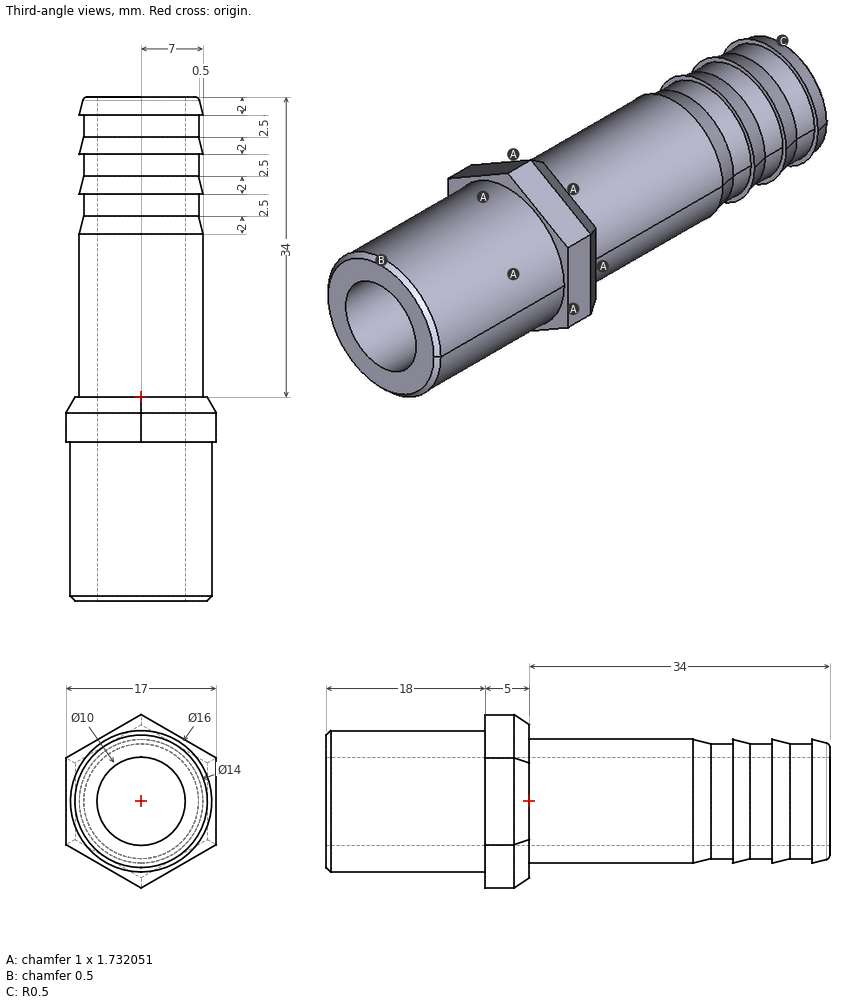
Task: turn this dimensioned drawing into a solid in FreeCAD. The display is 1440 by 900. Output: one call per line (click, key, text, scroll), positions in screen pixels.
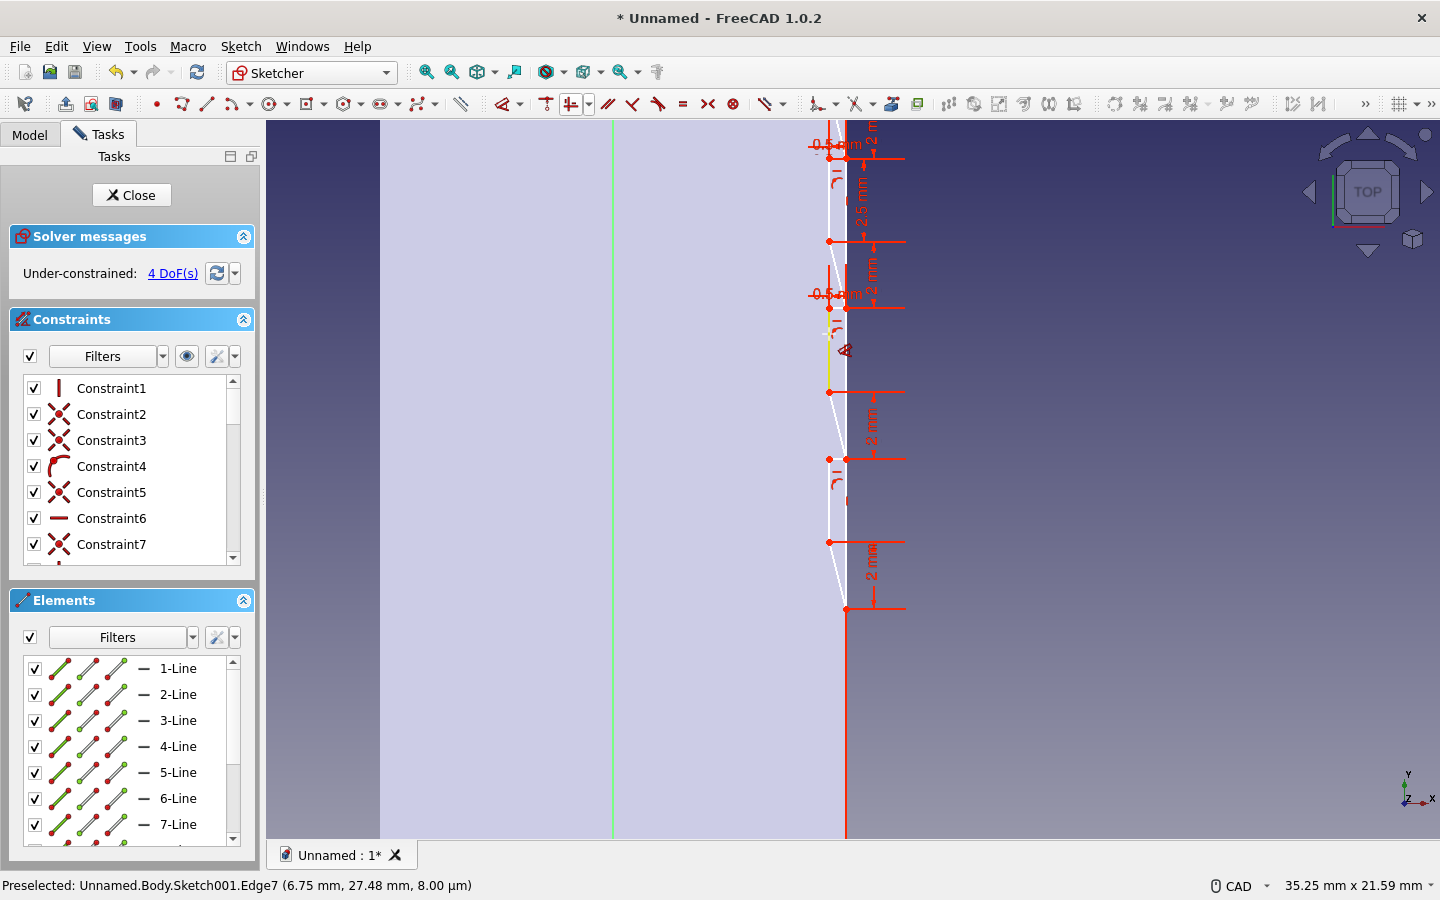
click(829, 334)
click(863, 350)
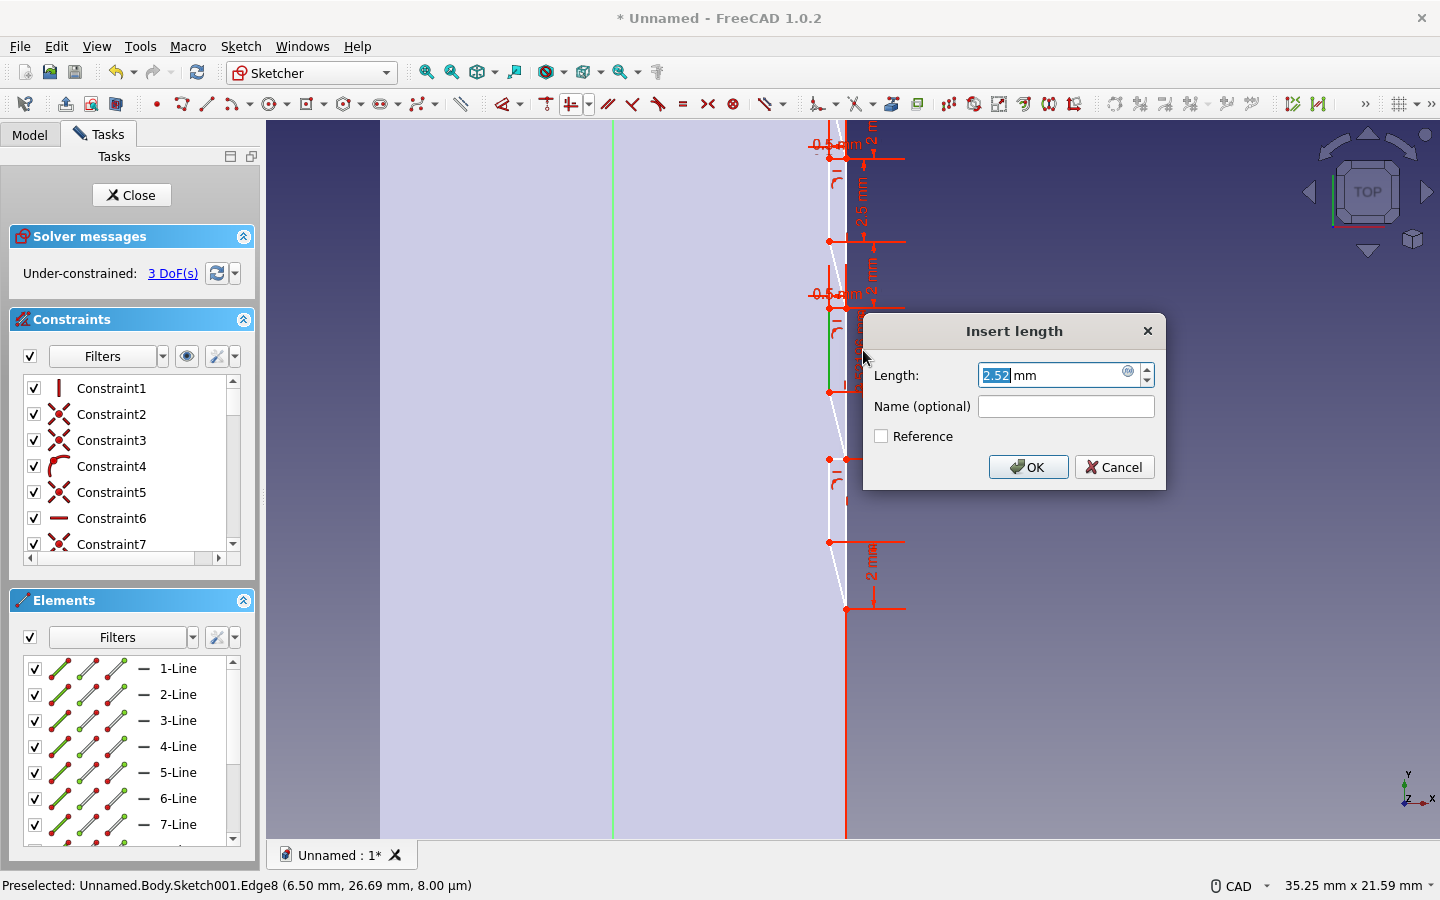
text(2.5)
key(Return)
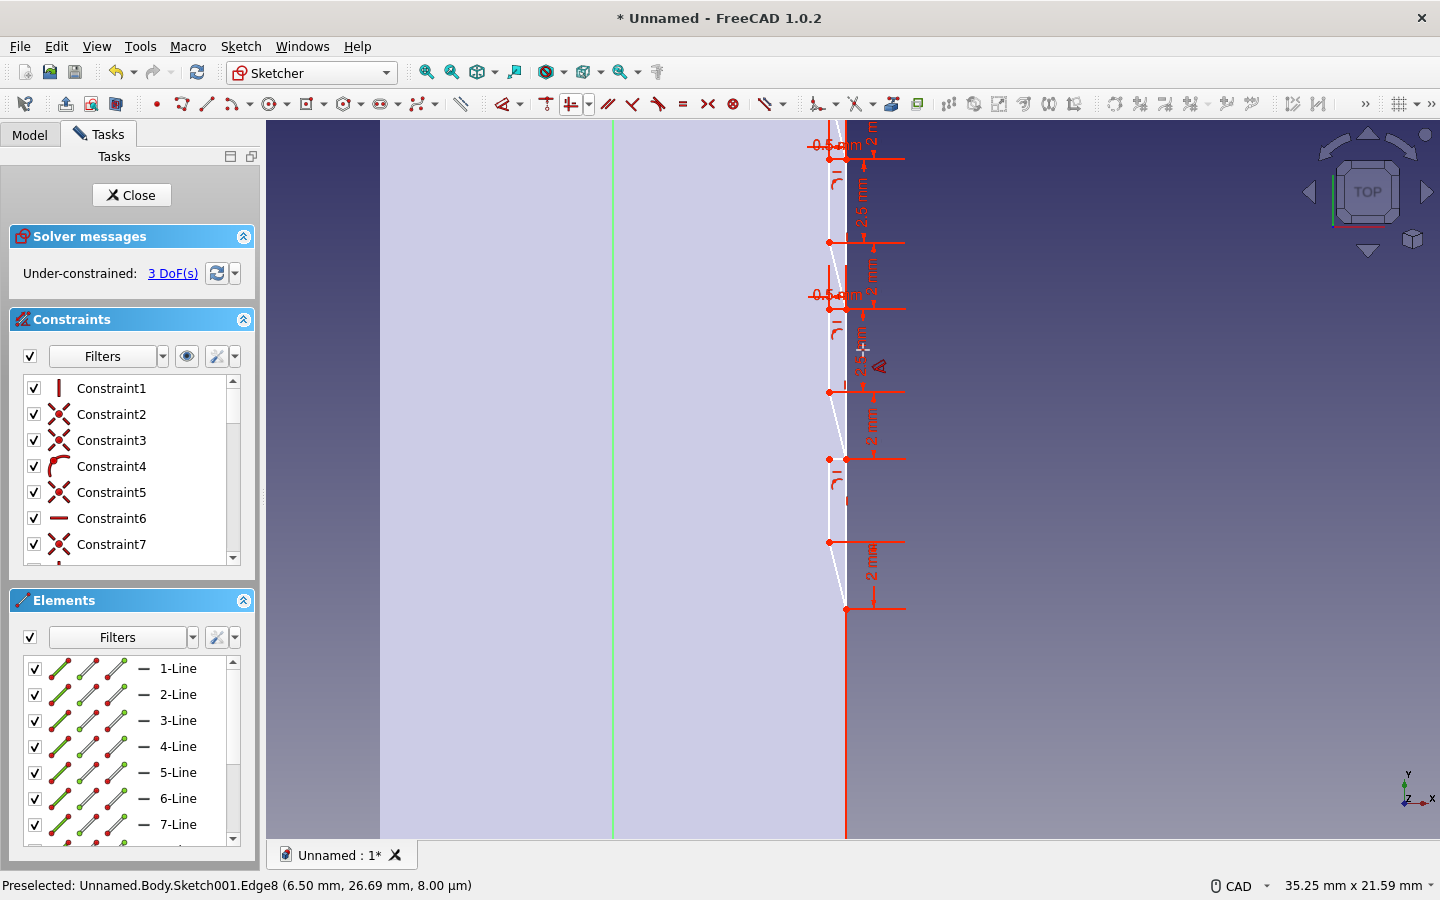
scroll(838, 459, up, 5)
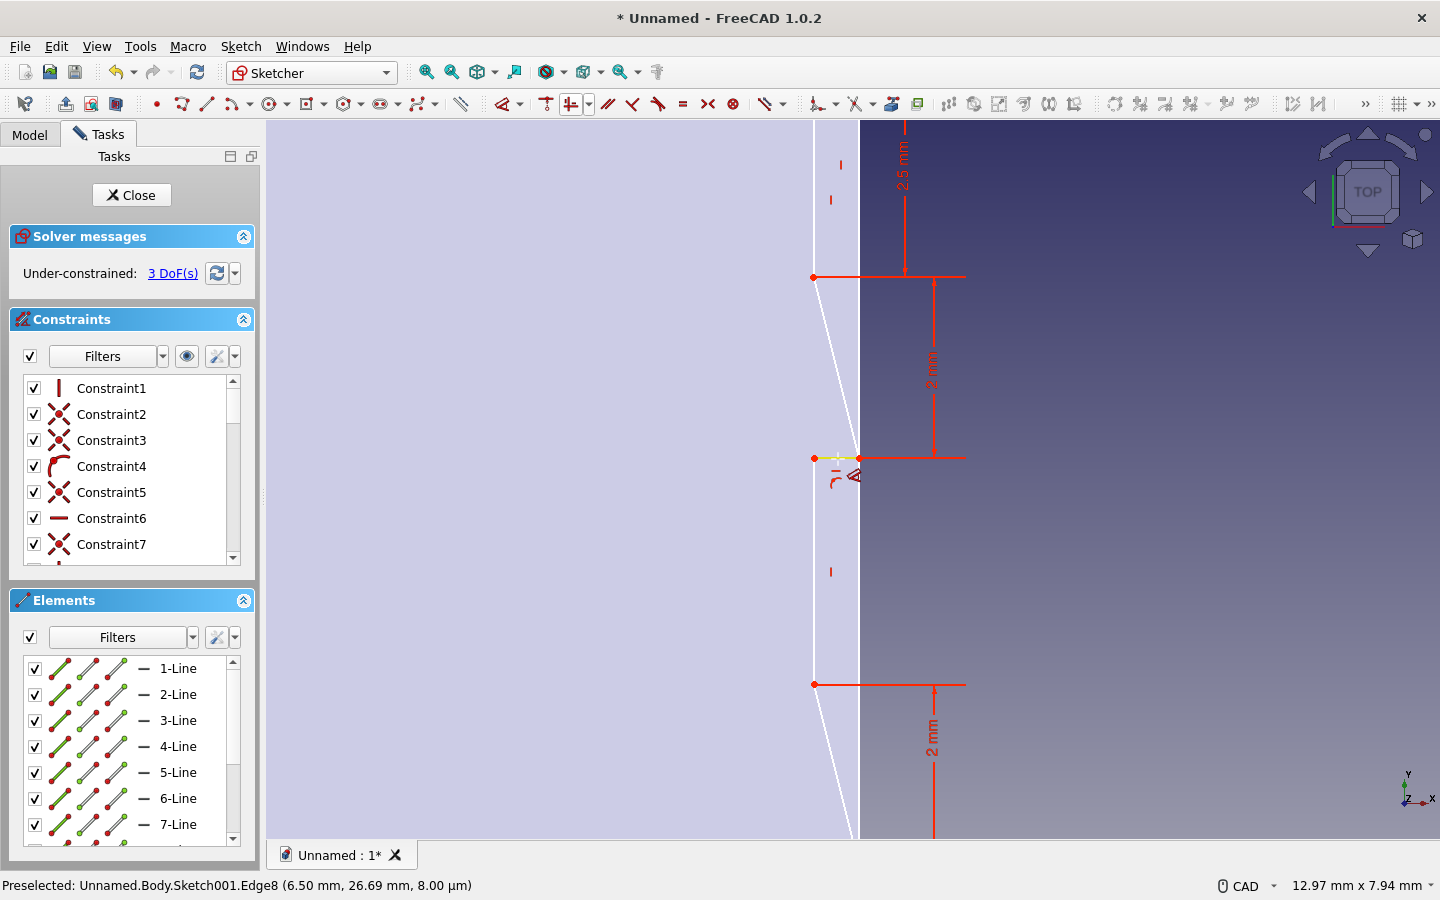
click(837, 458)
click(837, 424)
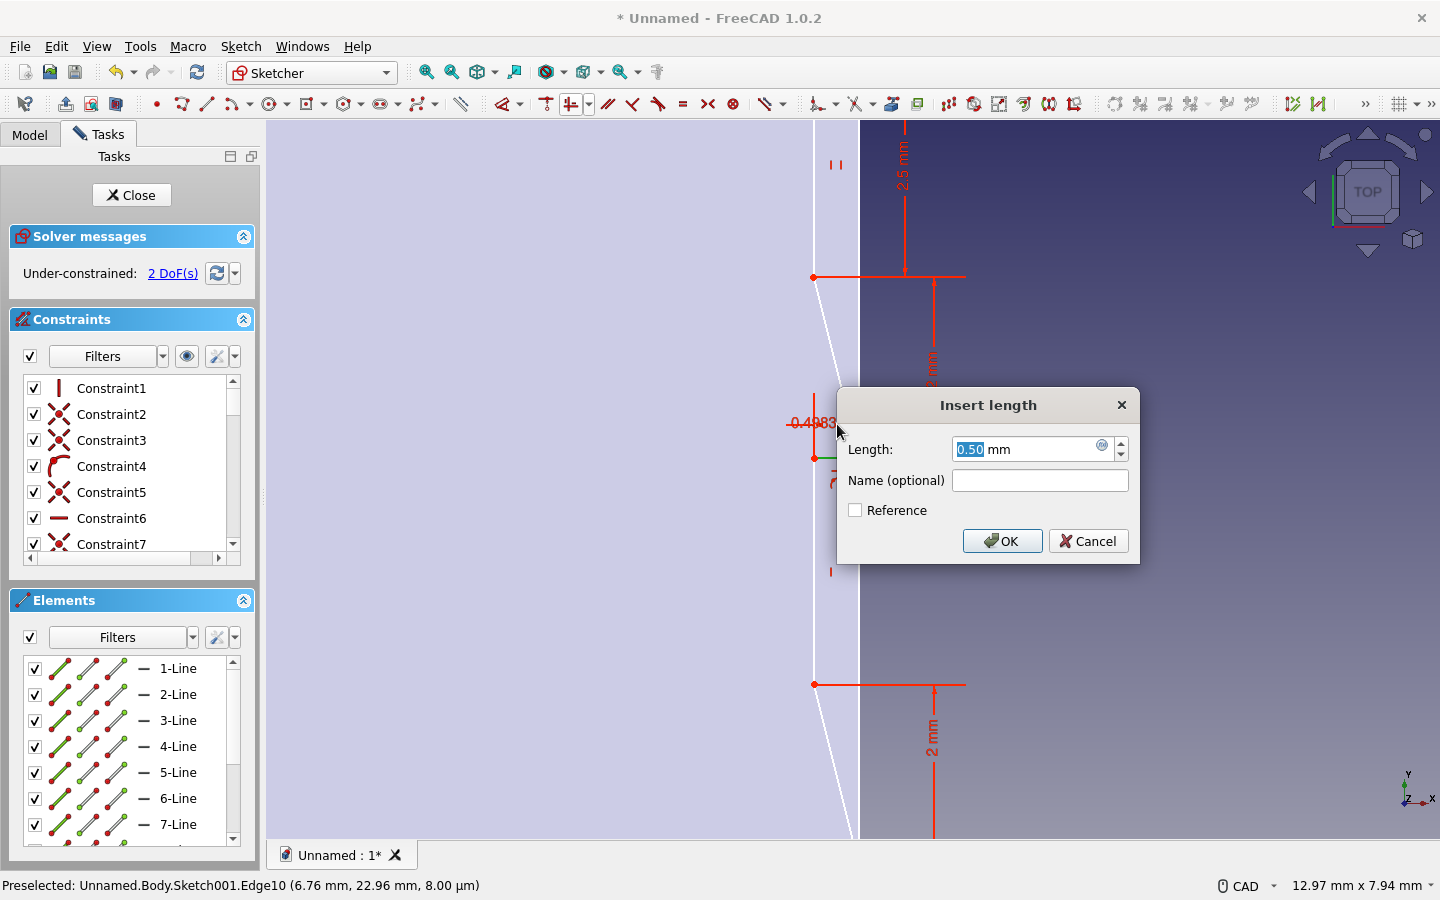
text(0.5)
key(Return)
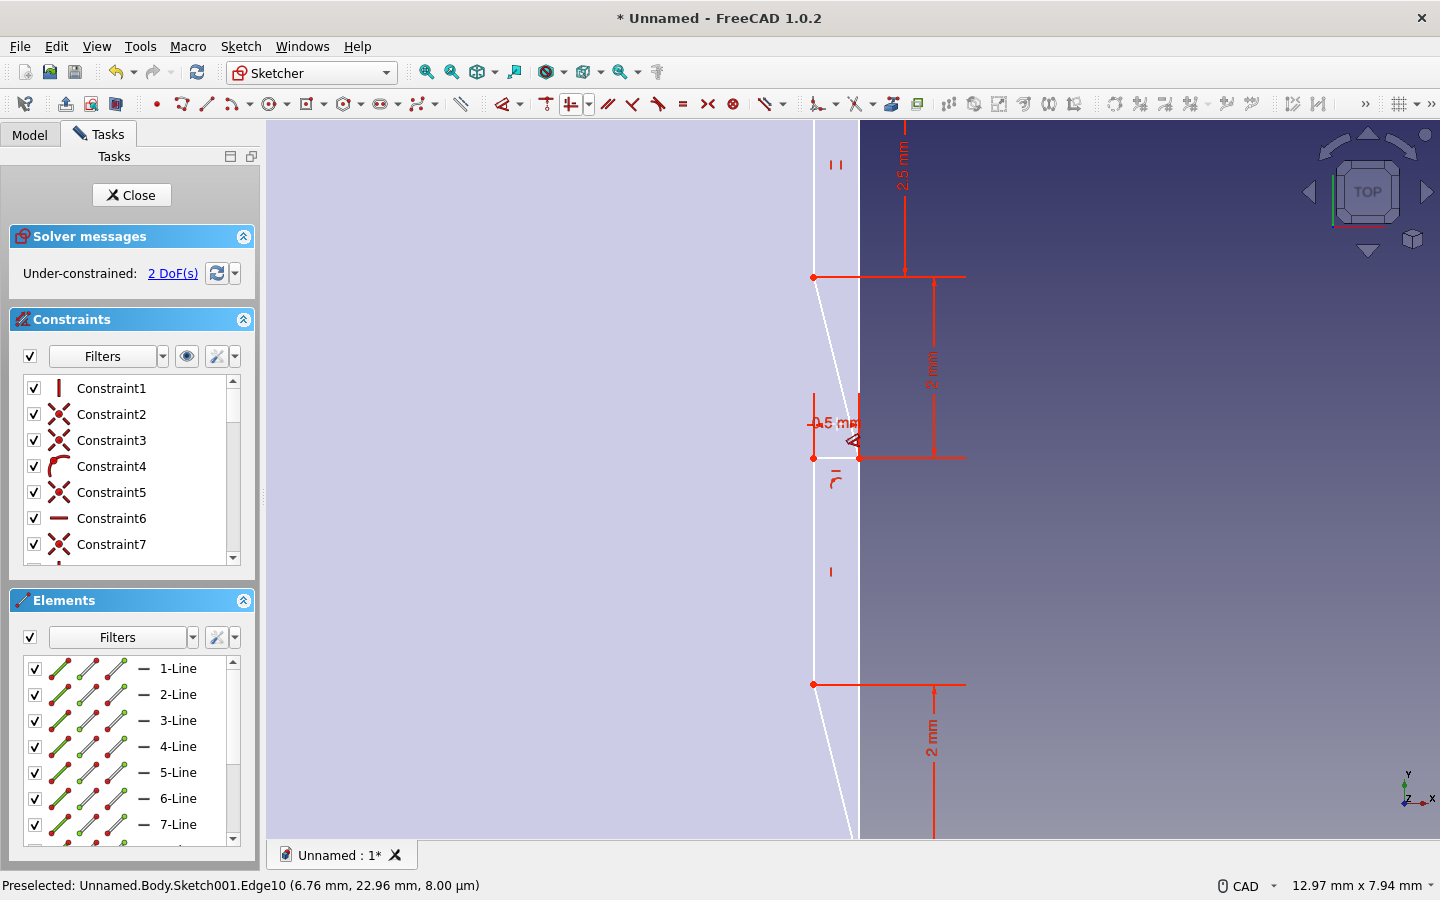
scroll(832, 377, down, 9)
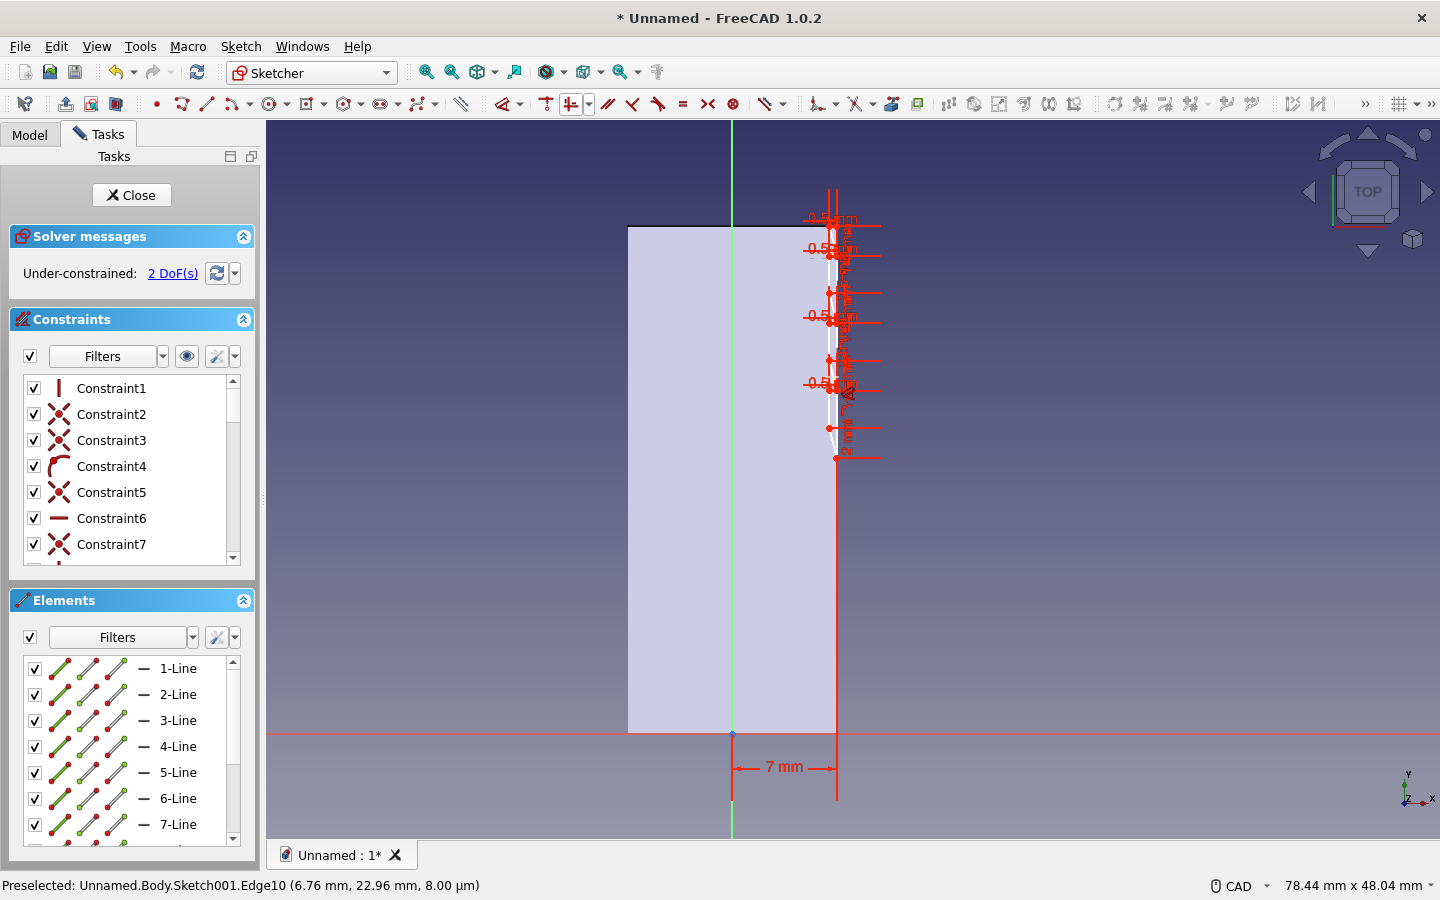
scroll(829, 402, up, 4)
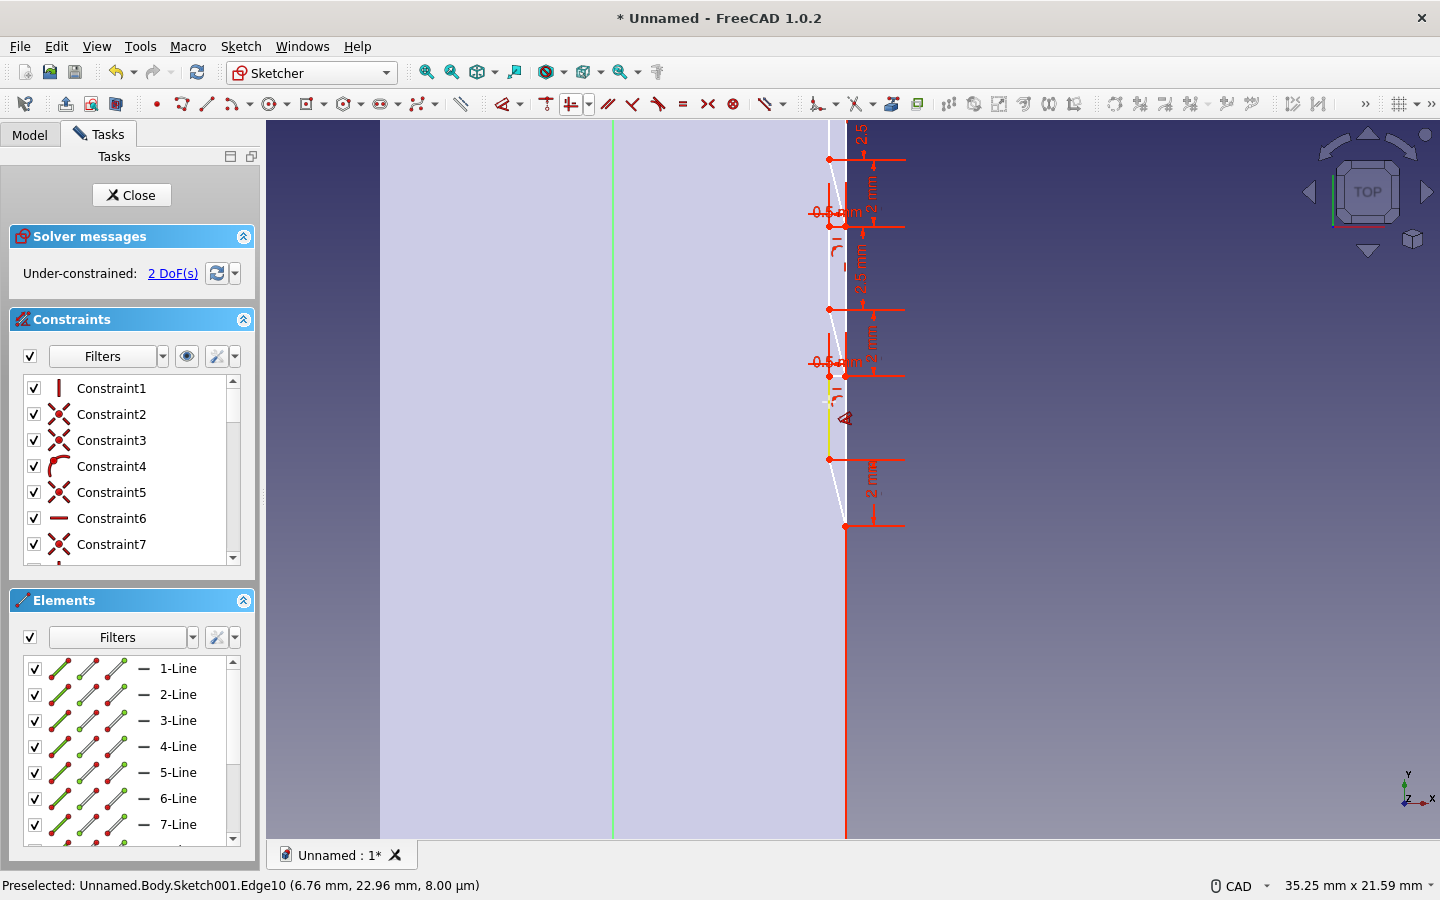
click(829, 401)
click(863, 418)